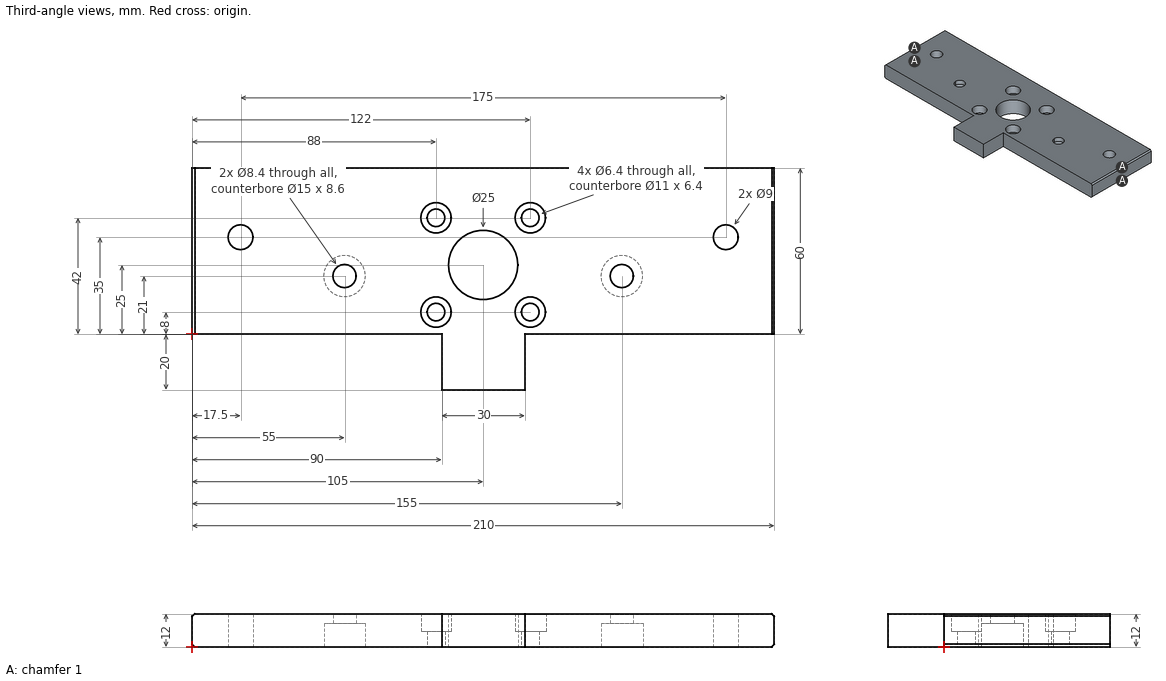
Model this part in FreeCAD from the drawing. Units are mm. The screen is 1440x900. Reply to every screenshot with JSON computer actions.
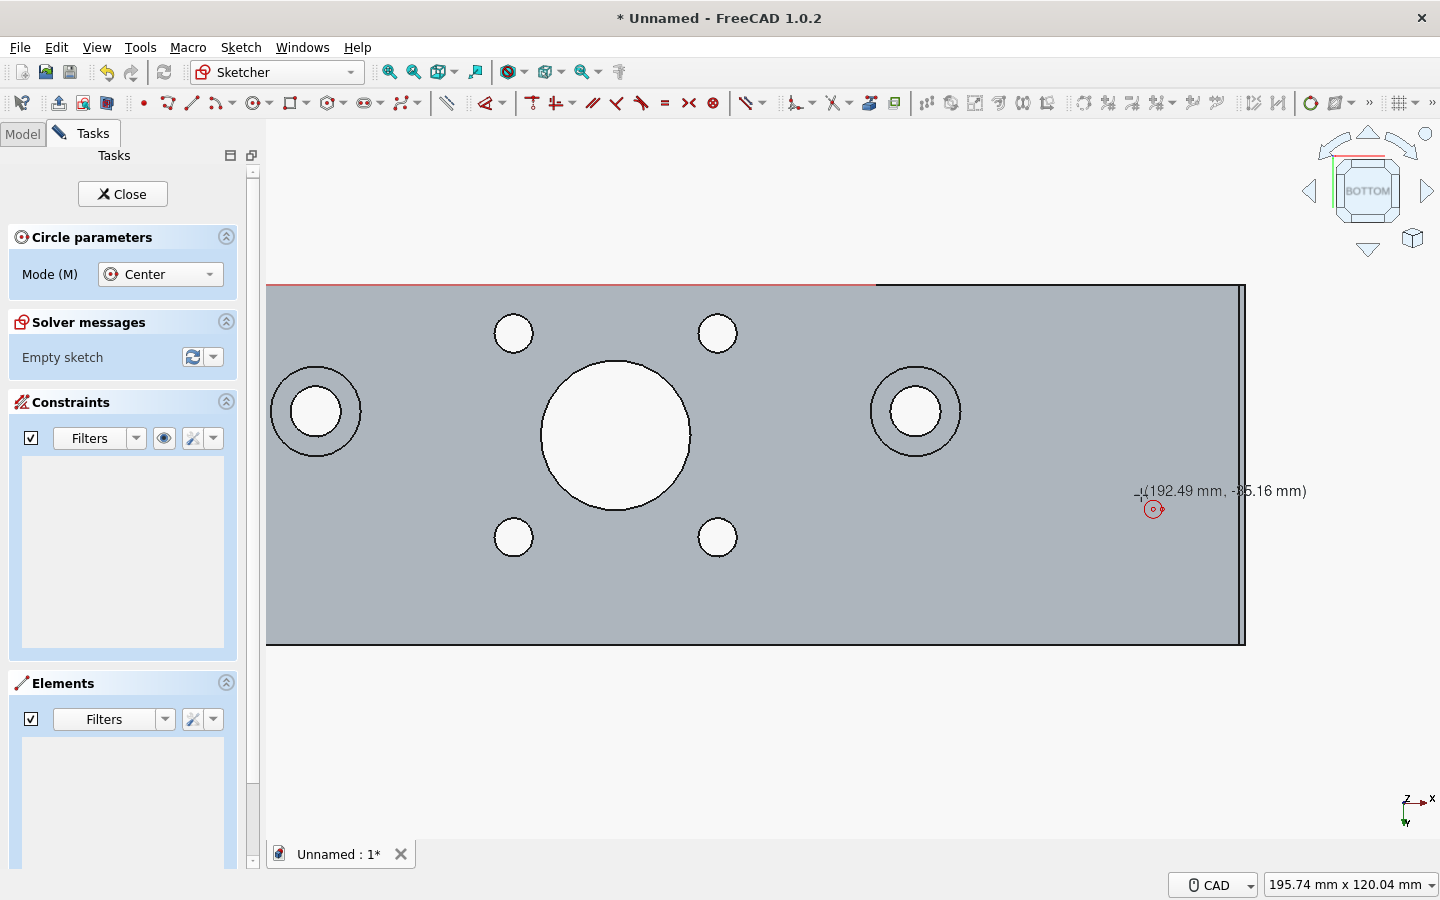
{"action": "left_click", "coordinate": [1140, 495]}
{"action": "left_click", "coordinate": [1160, 476]}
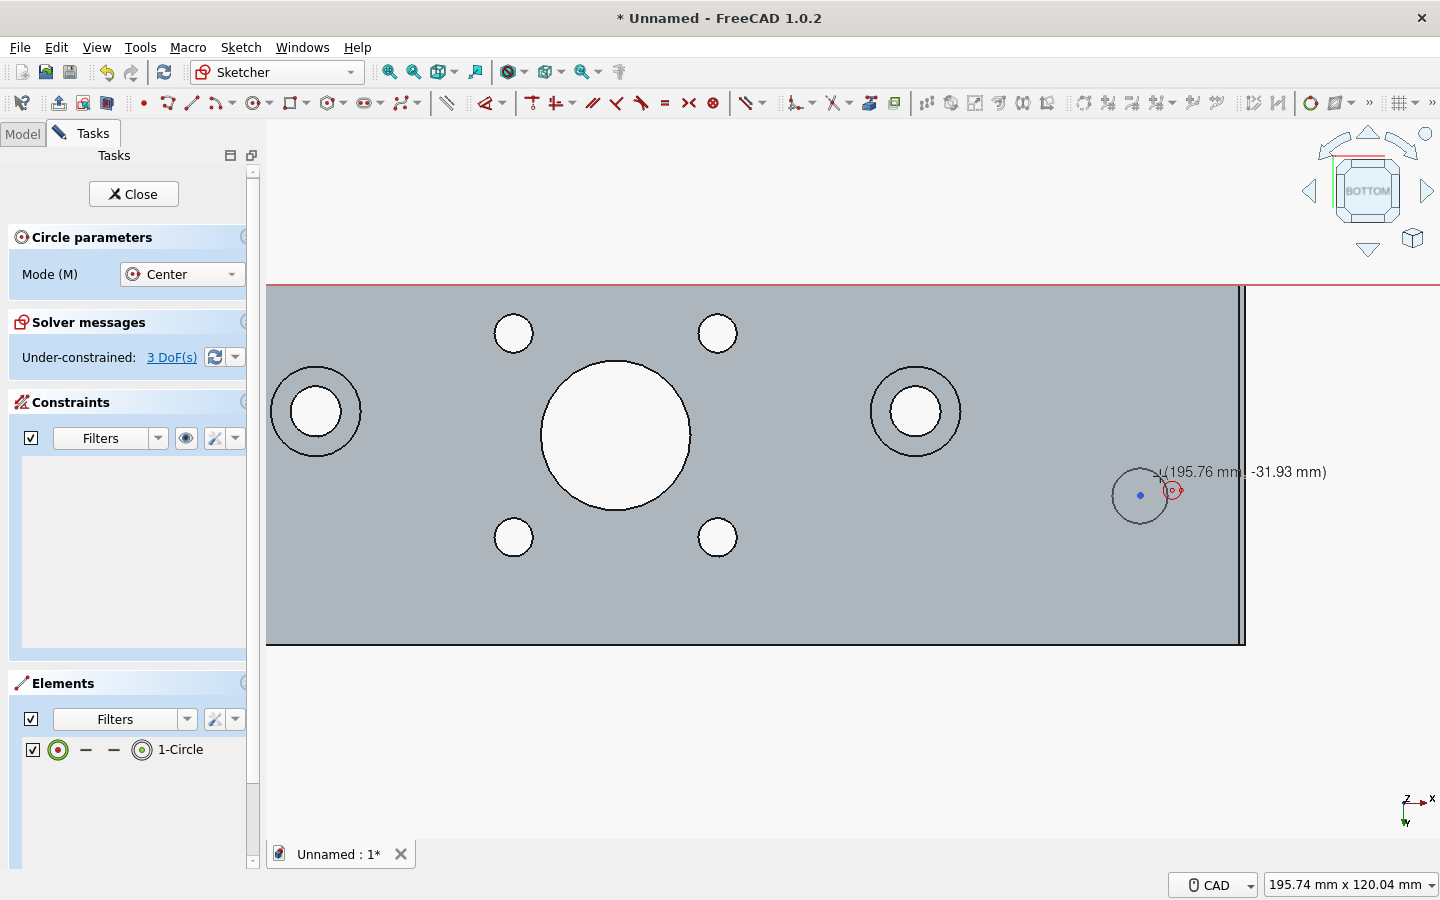
{"action": "scroll", "coordinate": [1037, 570], "scroll_direction": "down", "scroll_amount": 3}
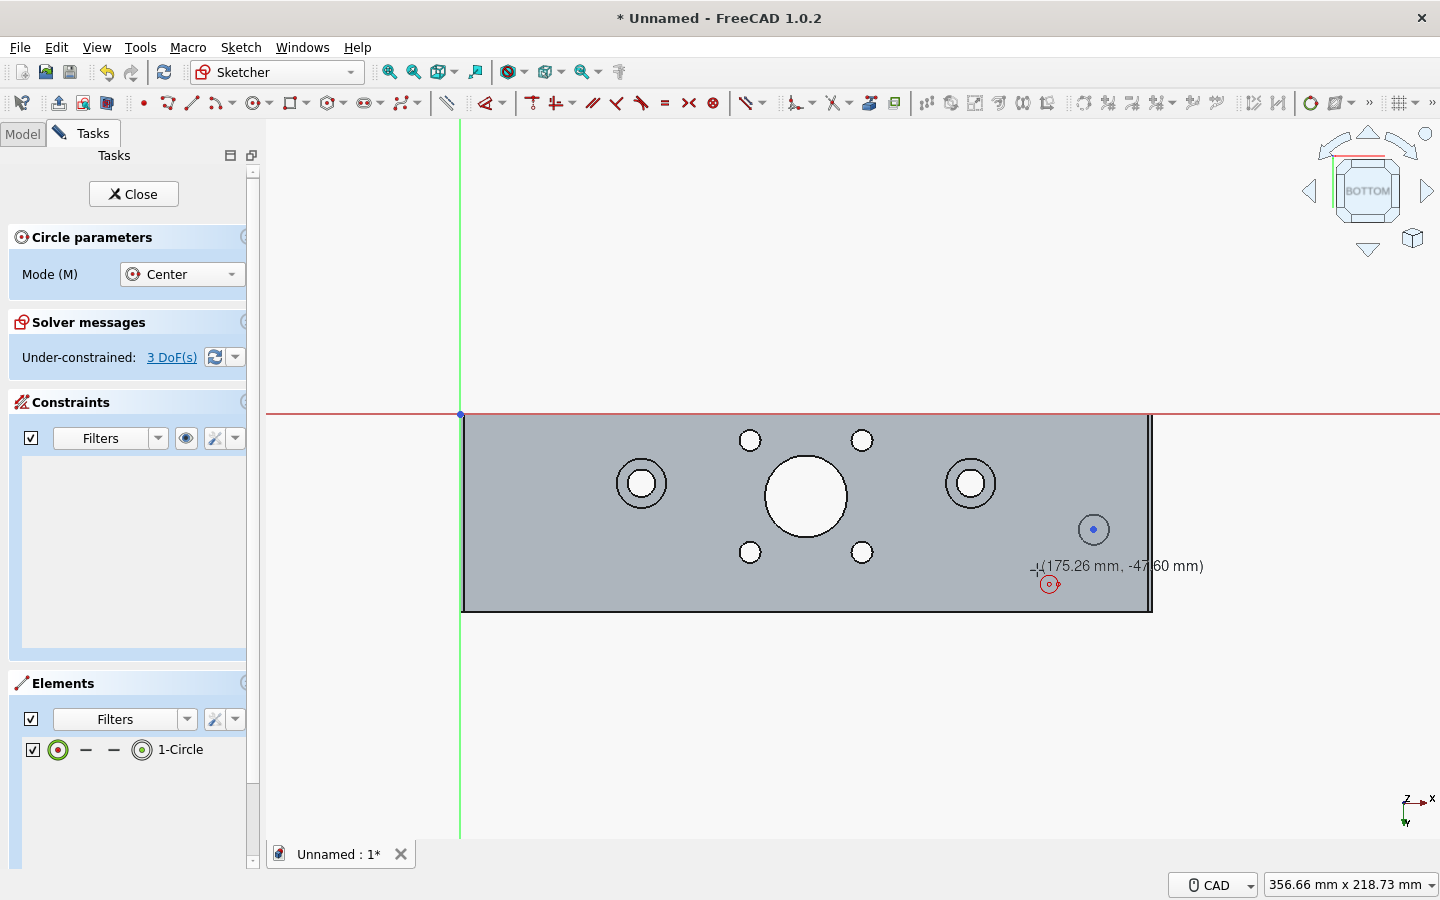
{"action": "scroll", "coordinate": [518, 529], "scroll_direction": "up", "scroll_amount": 3}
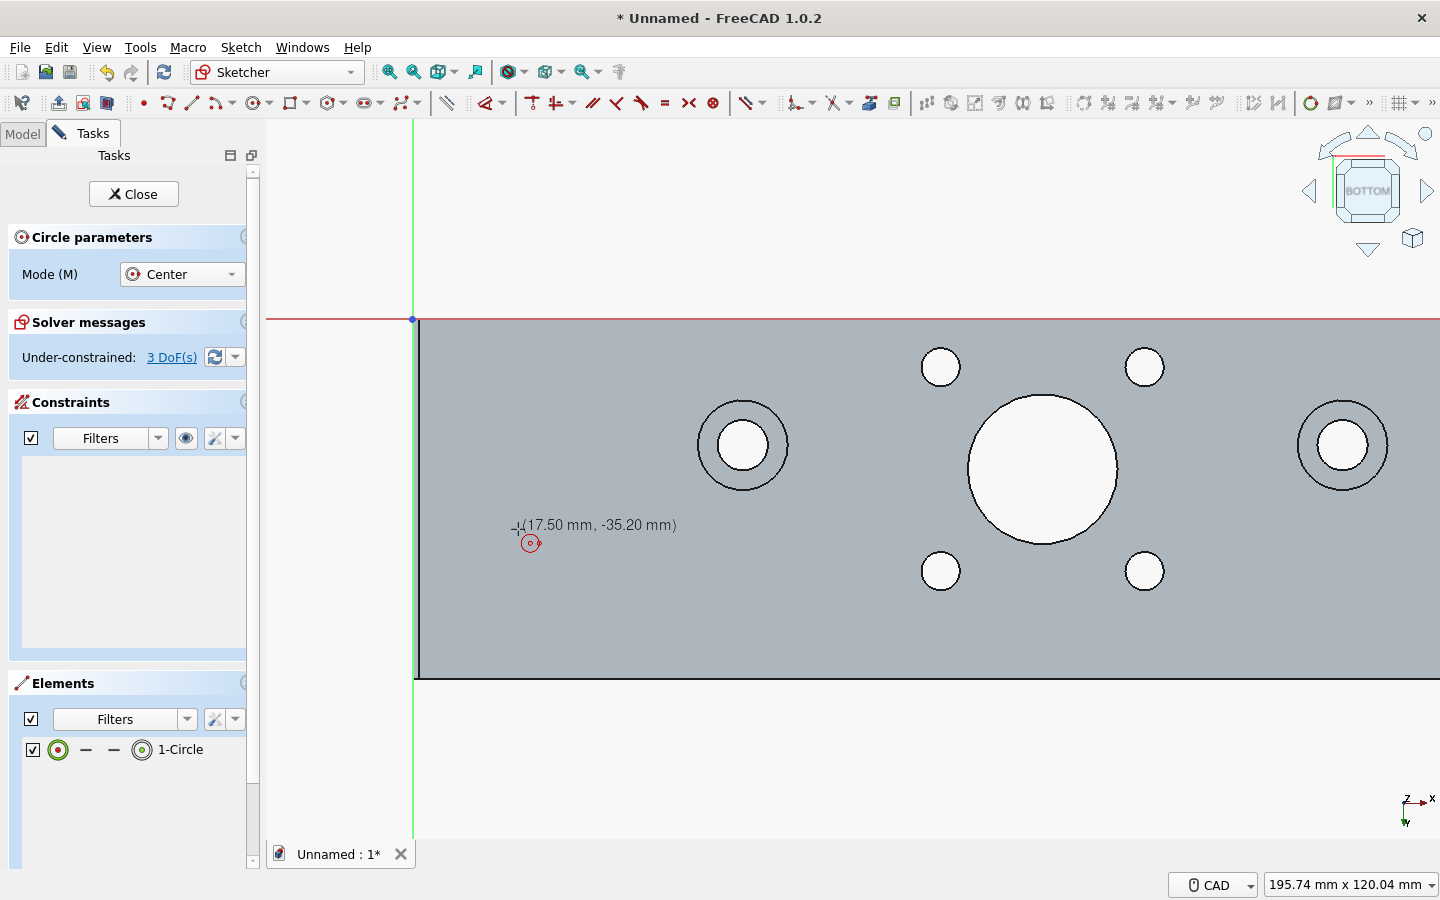
{"action": "left_click", "coordinate": [518, 529]}
{"action": "left_click", "coordinate": [537, 510]}
{"action": "key", "text": "Escape"}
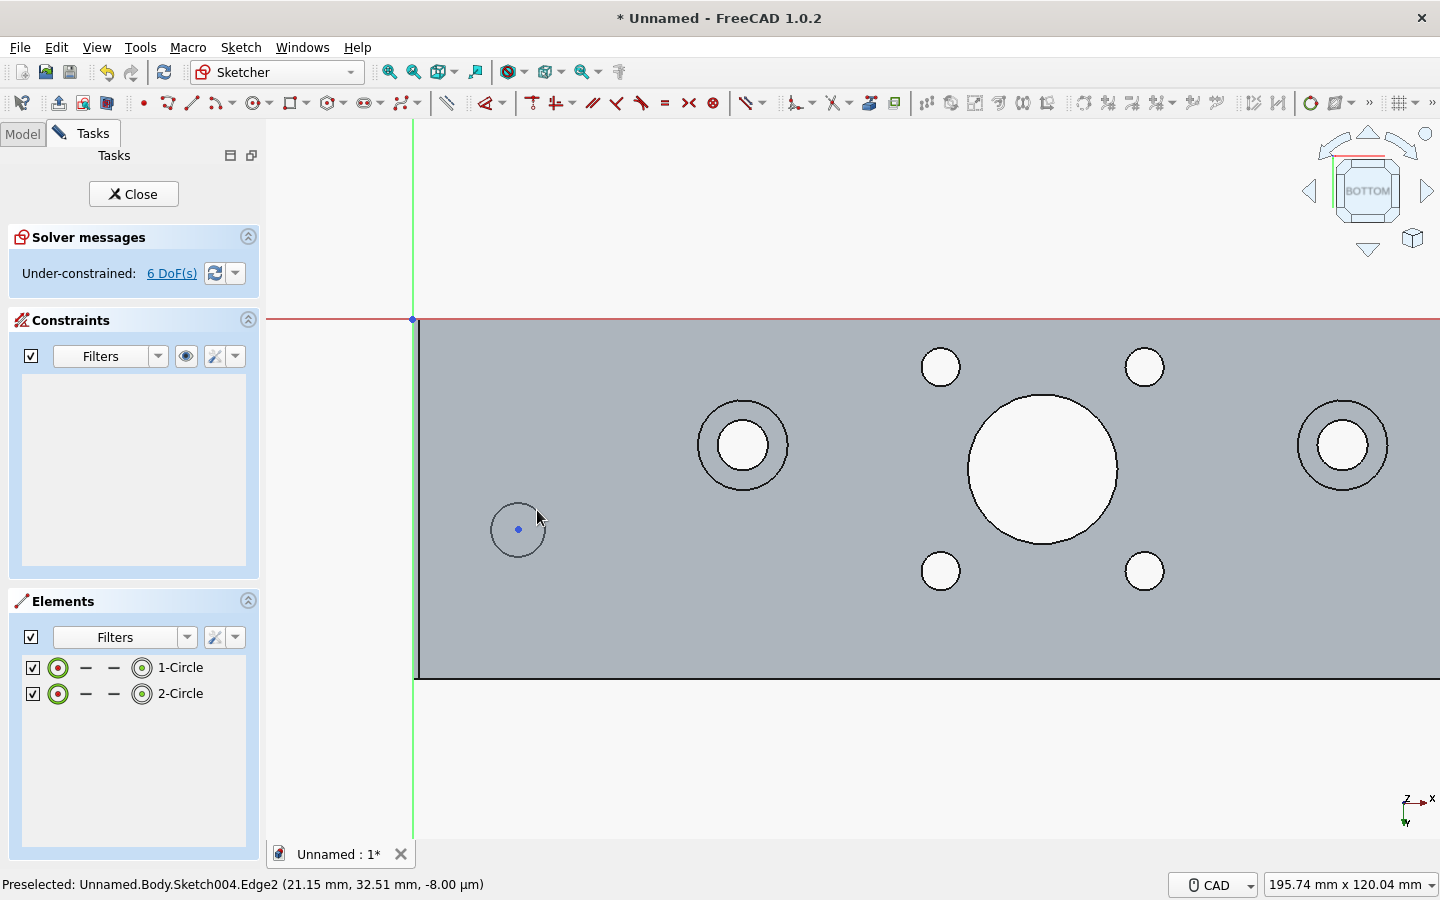
{"action": "scroll", "coordinate": [518, 529], "scroll_direction": "down", "scroll_amount": 3}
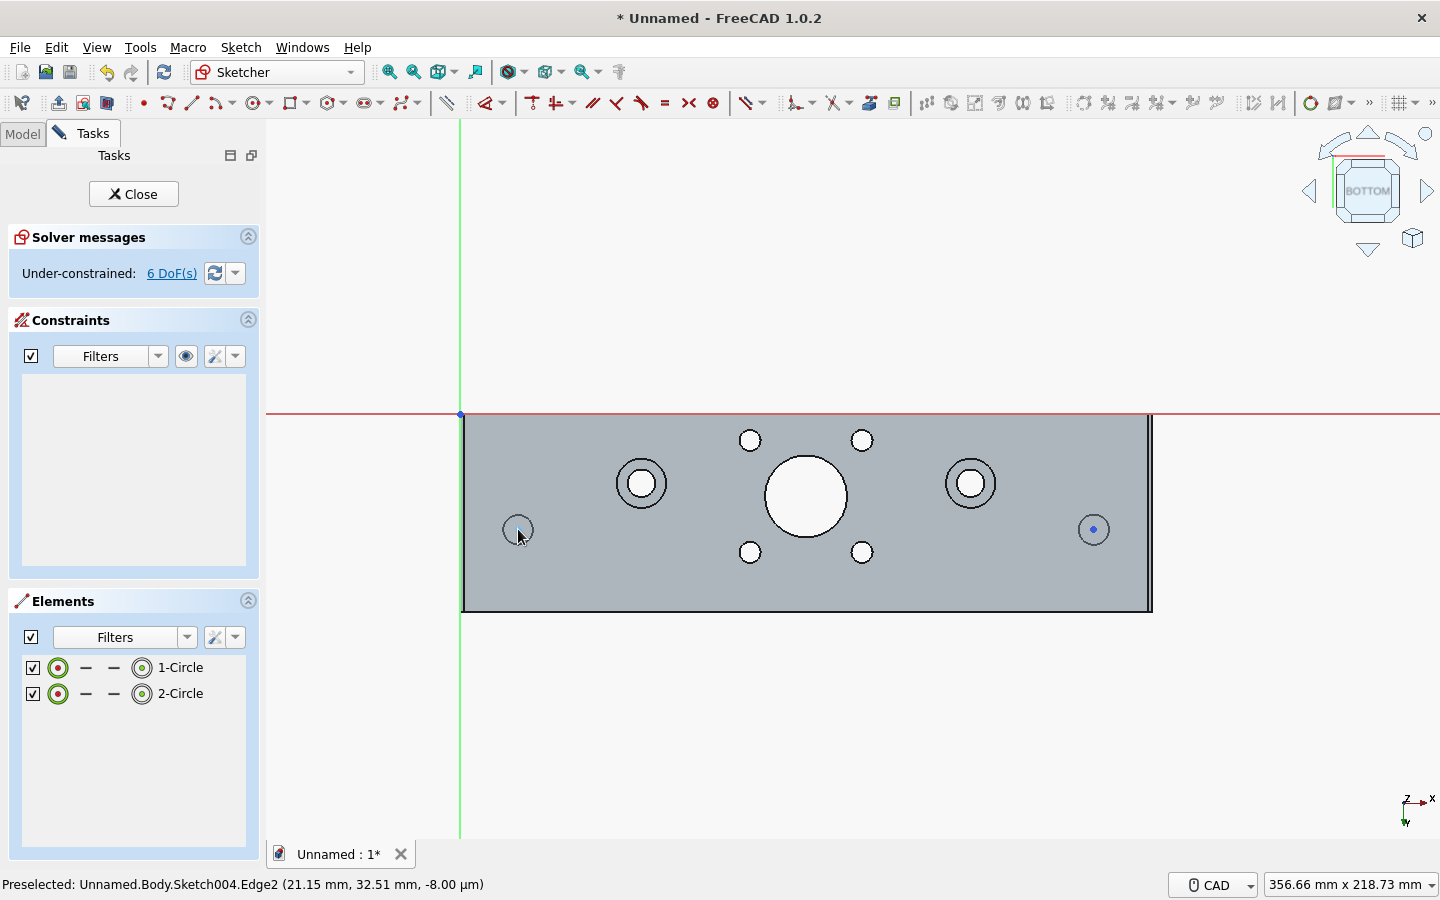
{"action": "left_click", "coordinate": [1104, 519]}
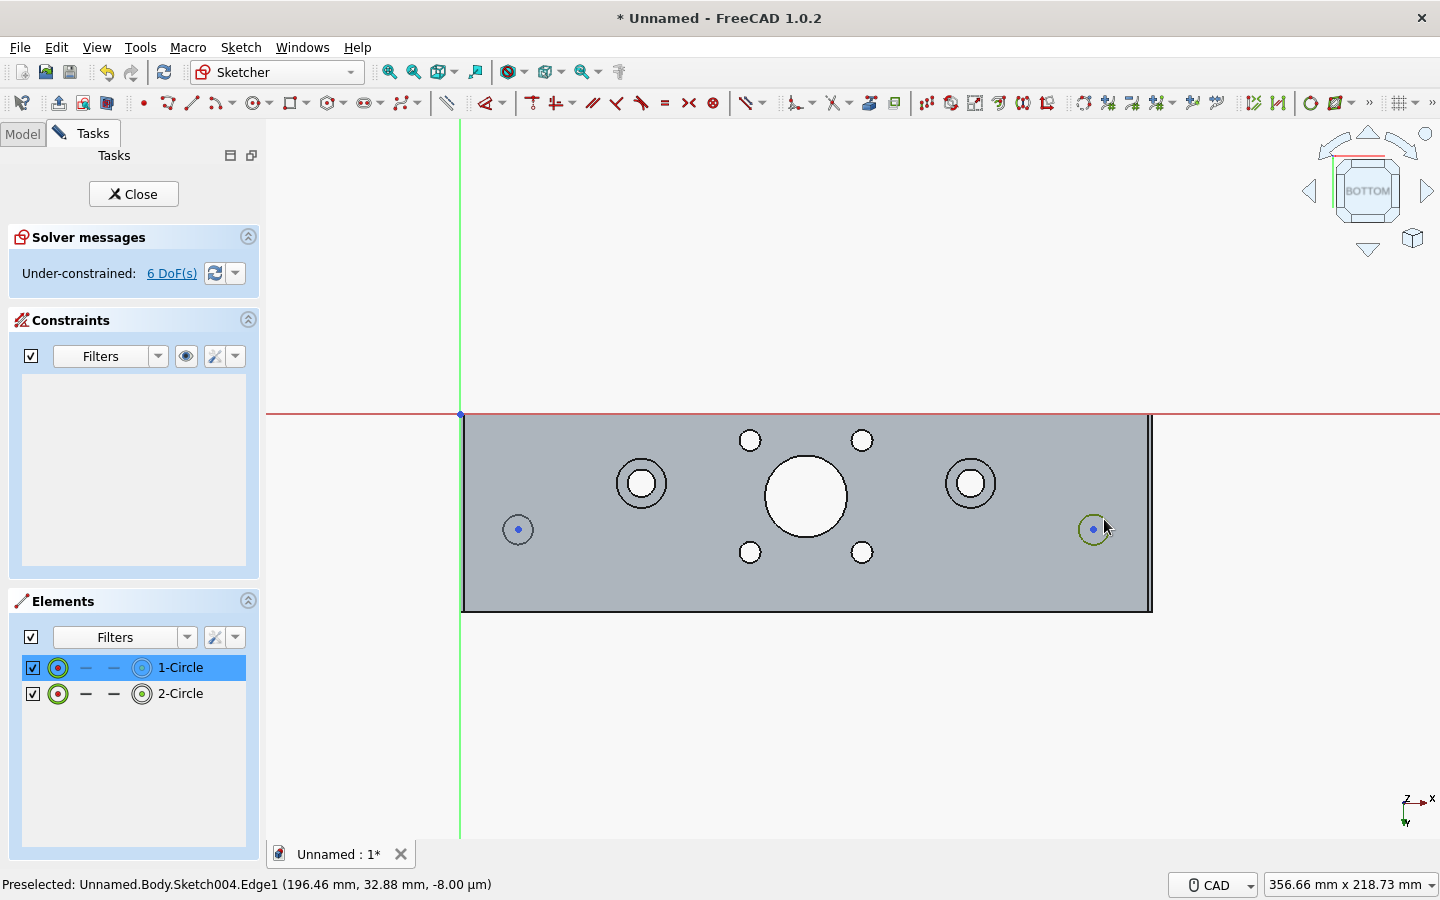
{"action": "left_click", "coordinate": [528, 519]}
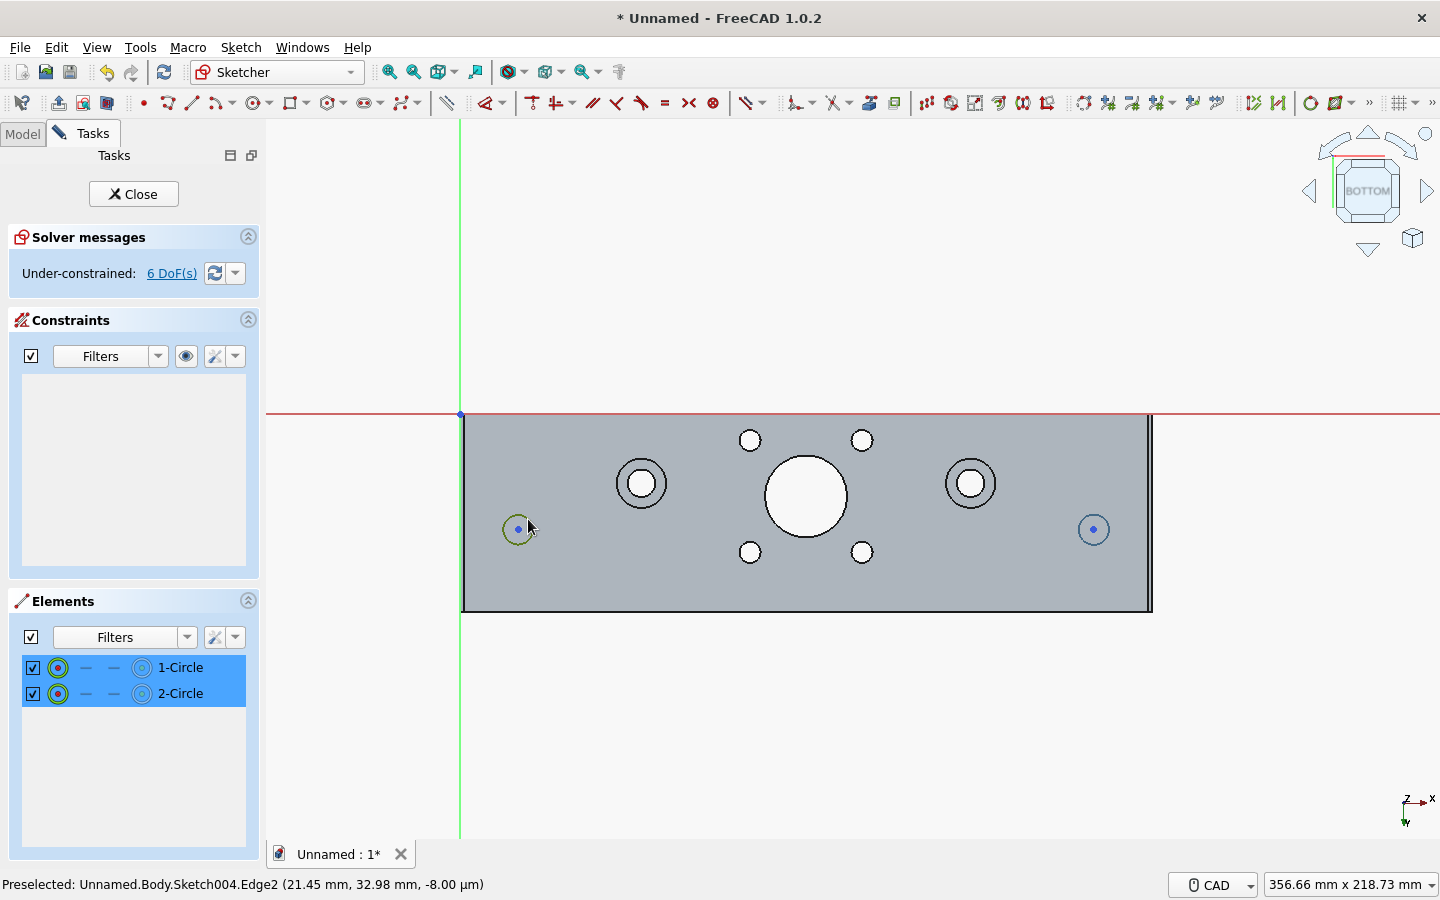
{"action": "key", "text": "e"}